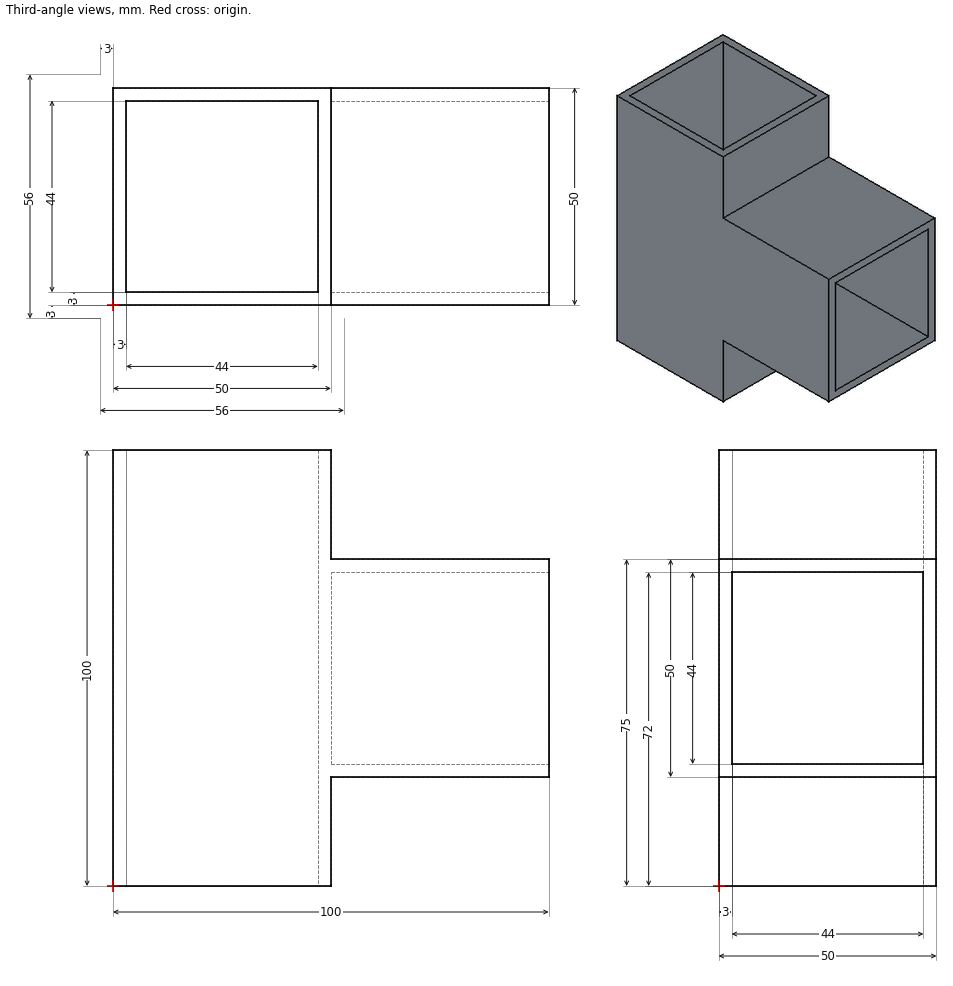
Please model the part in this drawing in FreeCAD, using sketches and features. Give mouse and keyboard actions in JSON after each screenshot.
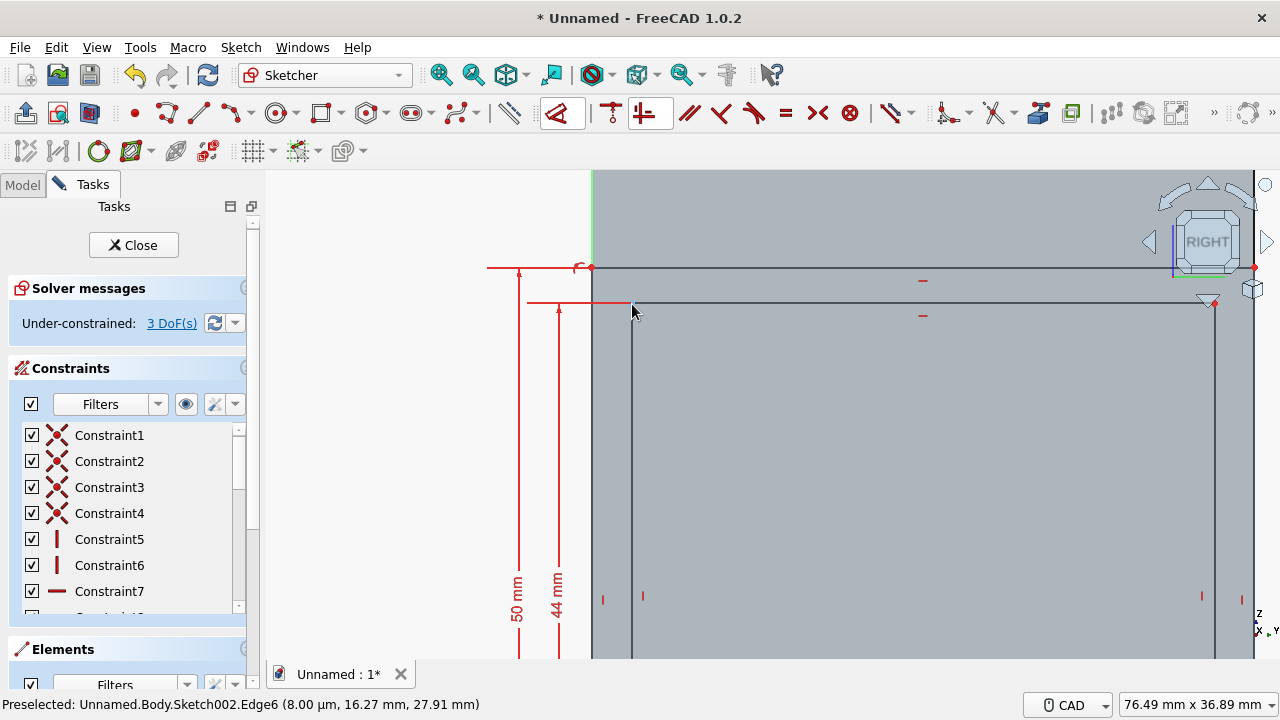
{"action": "left_click", "coordinate": [632, 303]}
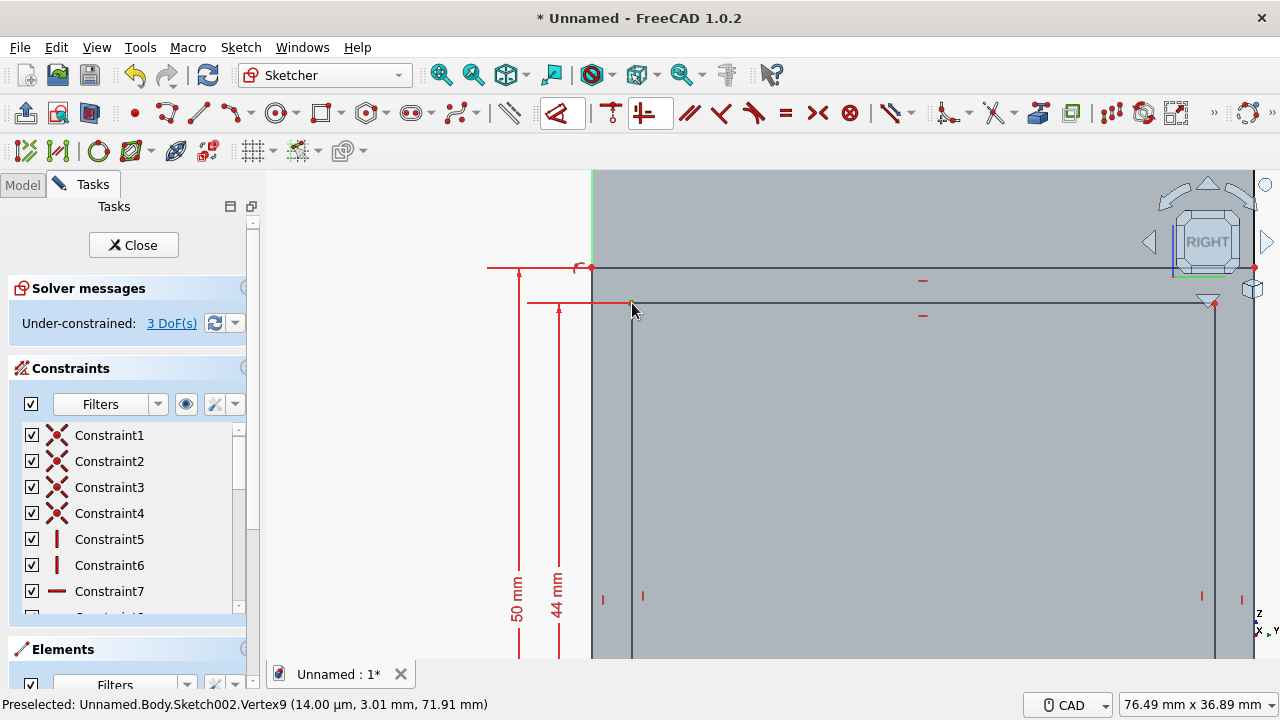
{"action": "key", "text": "l"}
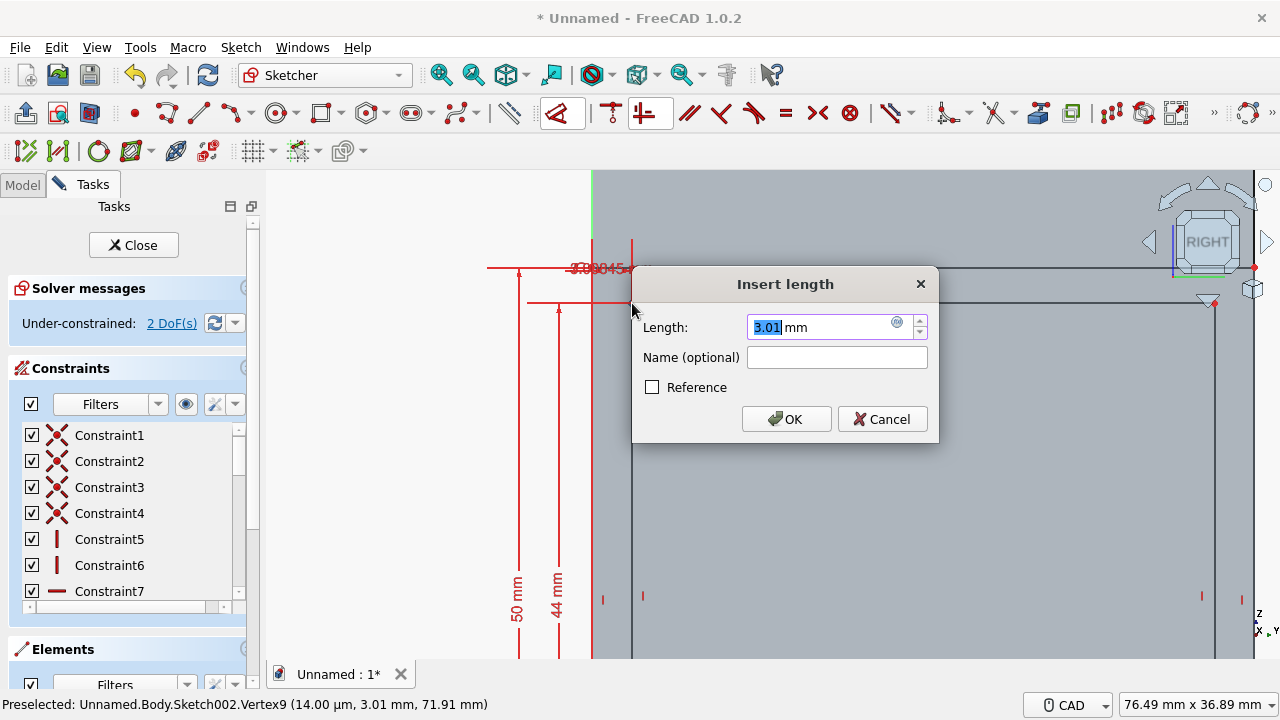
{"action": "type", "text": "3"}
{"action": "key", "text": "Return"}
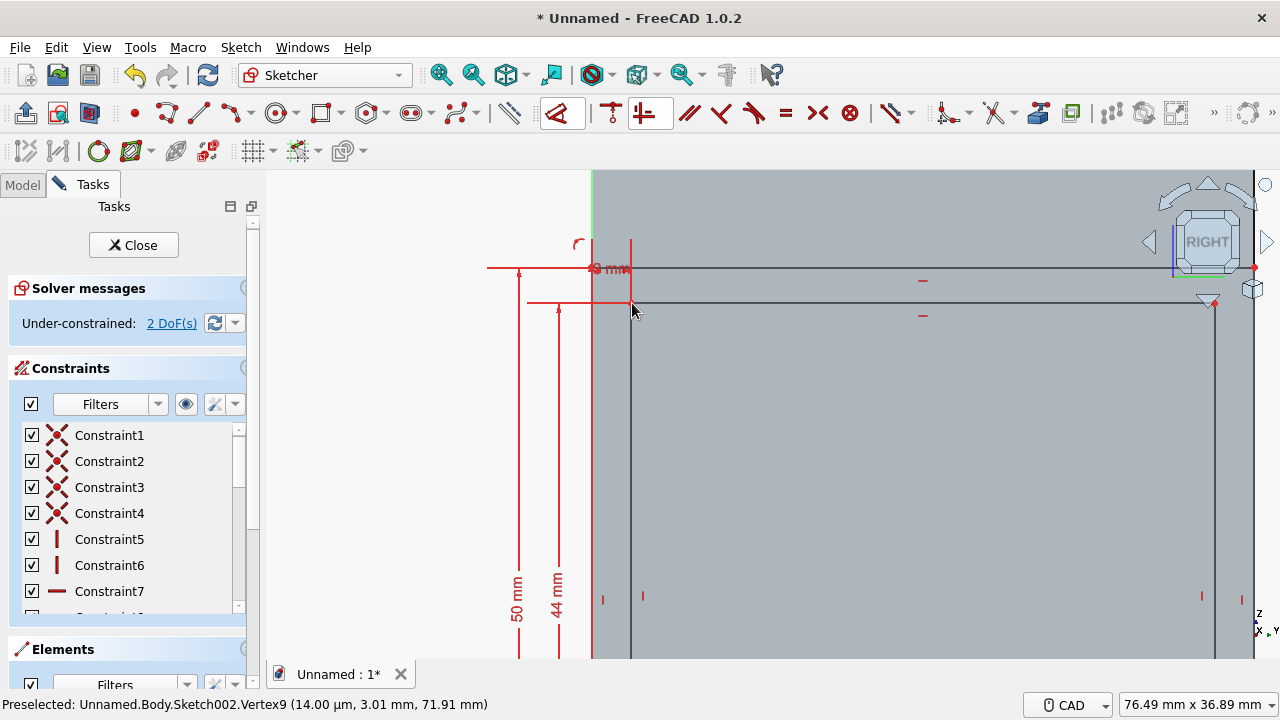
{"action": "scroll", "coordinate": [610, 266], "scroll_direction": "down", "scroll_amount": 6}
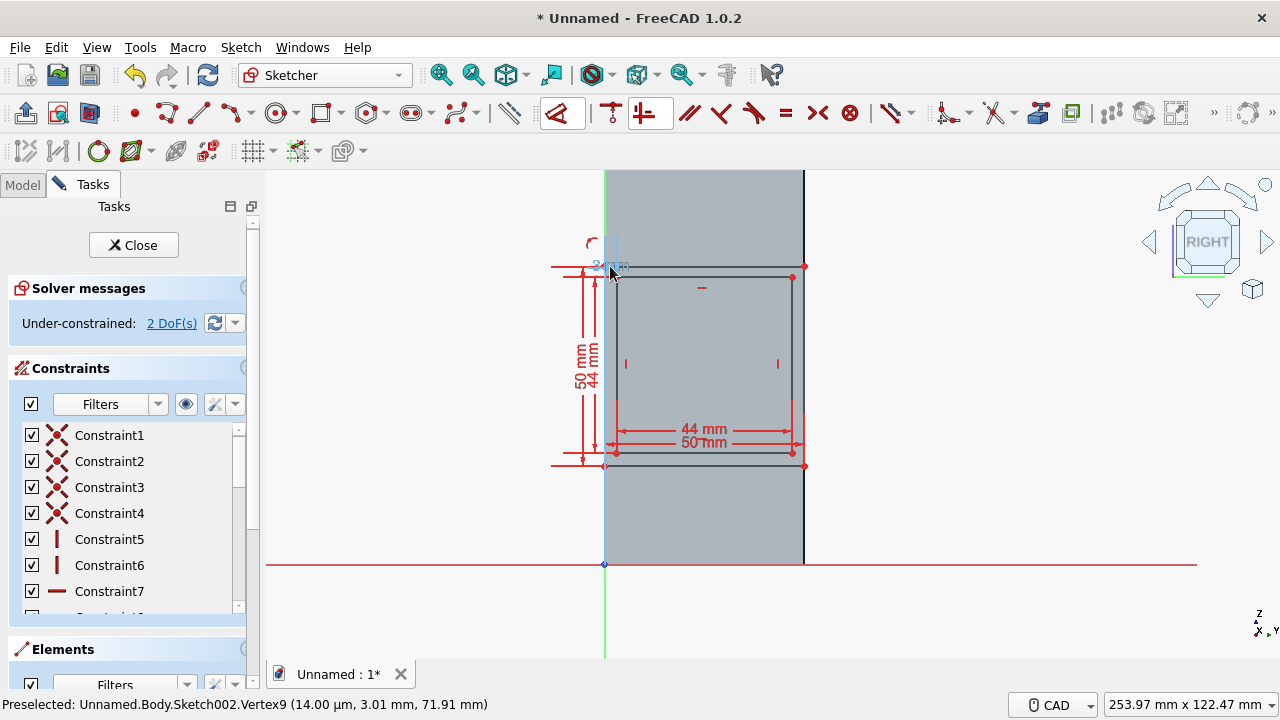
{"action": "left_click", "coordinate": [605, 267]}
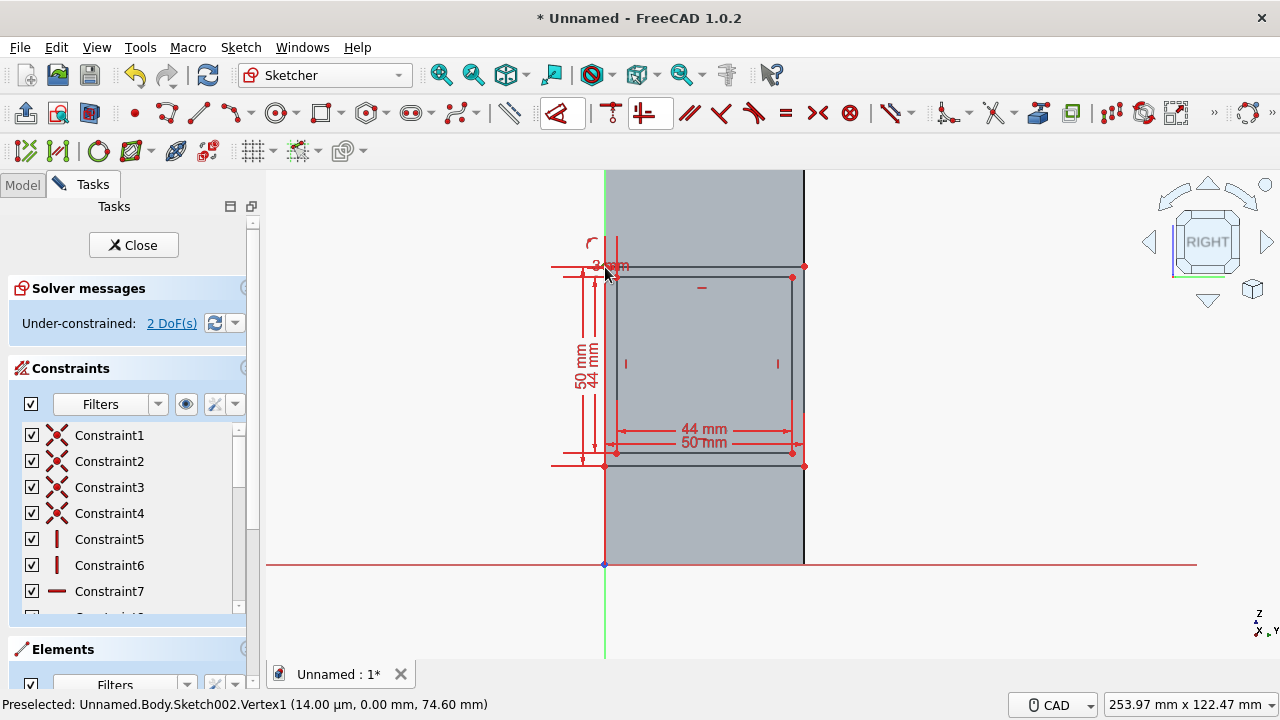
{"action": "key", "text": "i"}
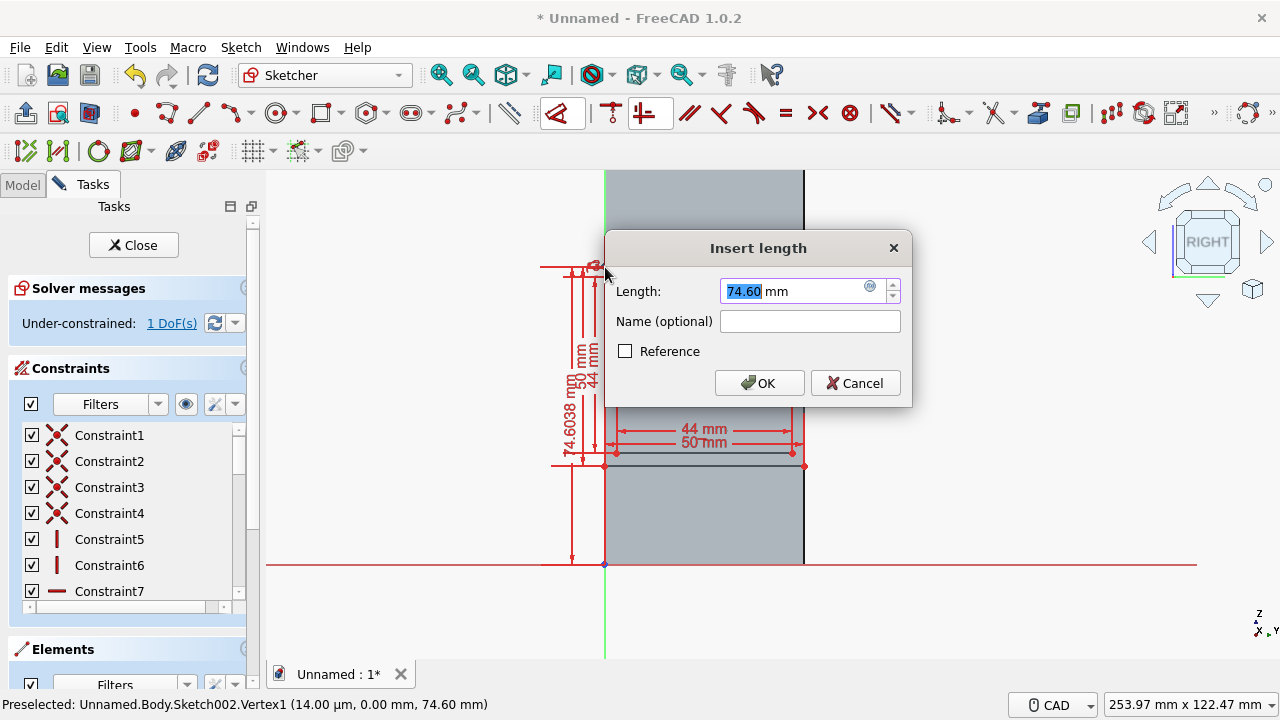
{"action": "type", "text": "75"}
{"action": "key", "text": "Return"}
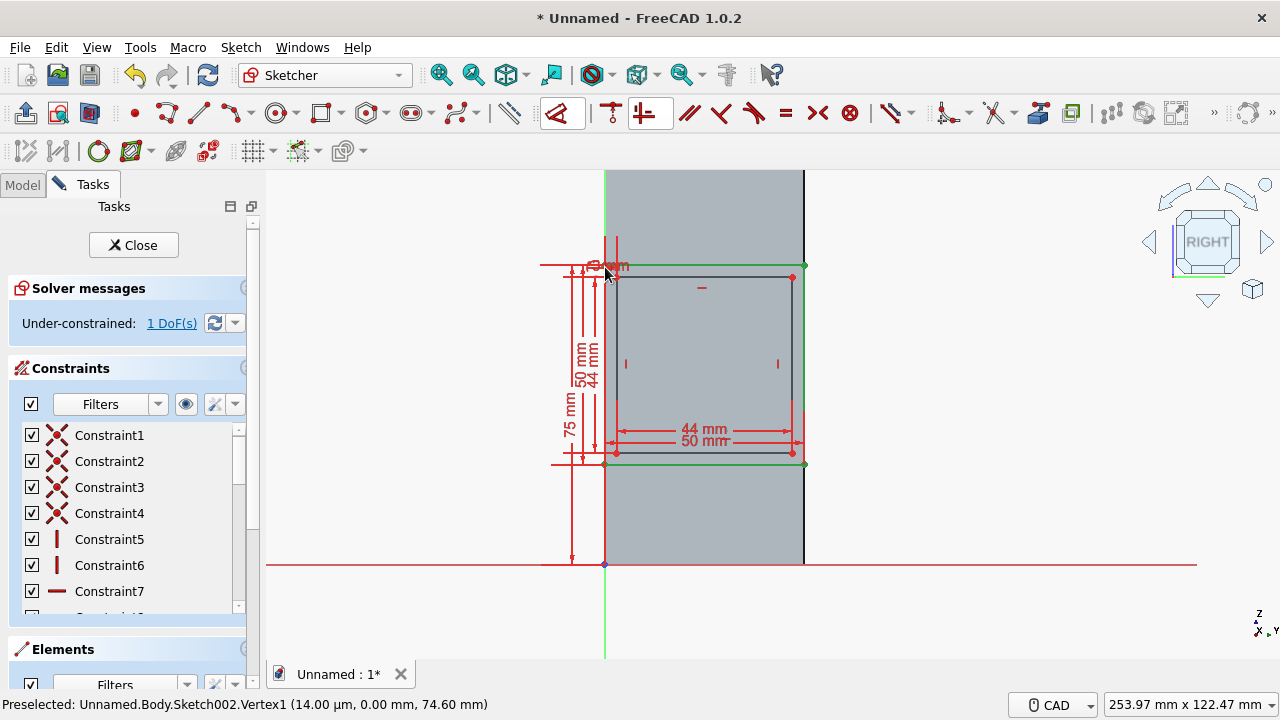
{"action": "left_click", "coordinate": [617, 277]}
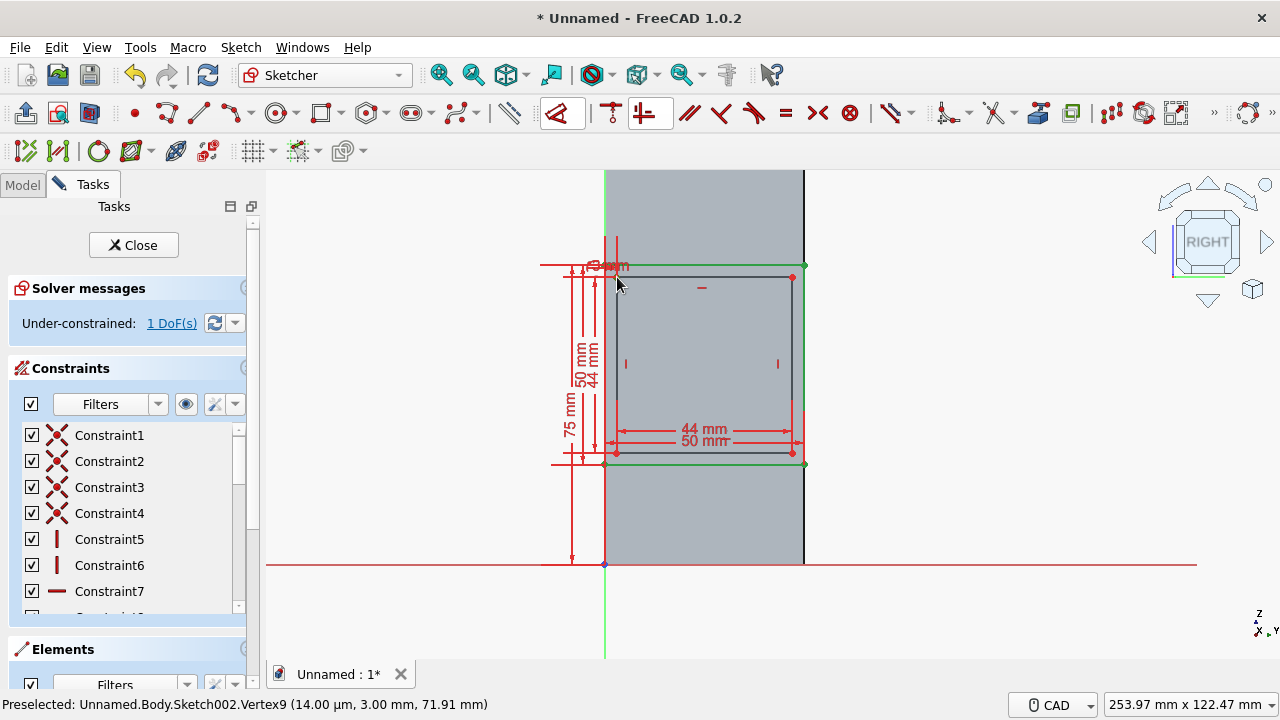
{"action": "key", "text": "i"}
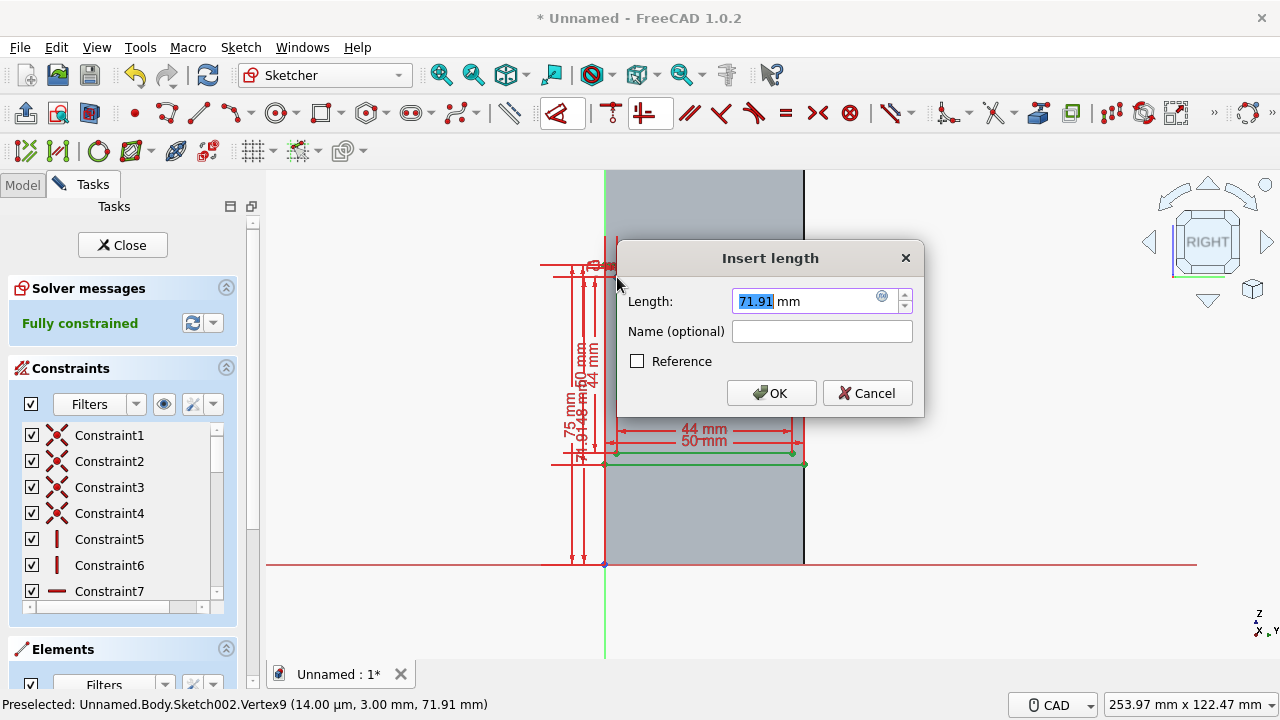
{"action": "type", "text": "72"}
{"action": "key", "text": "Return"}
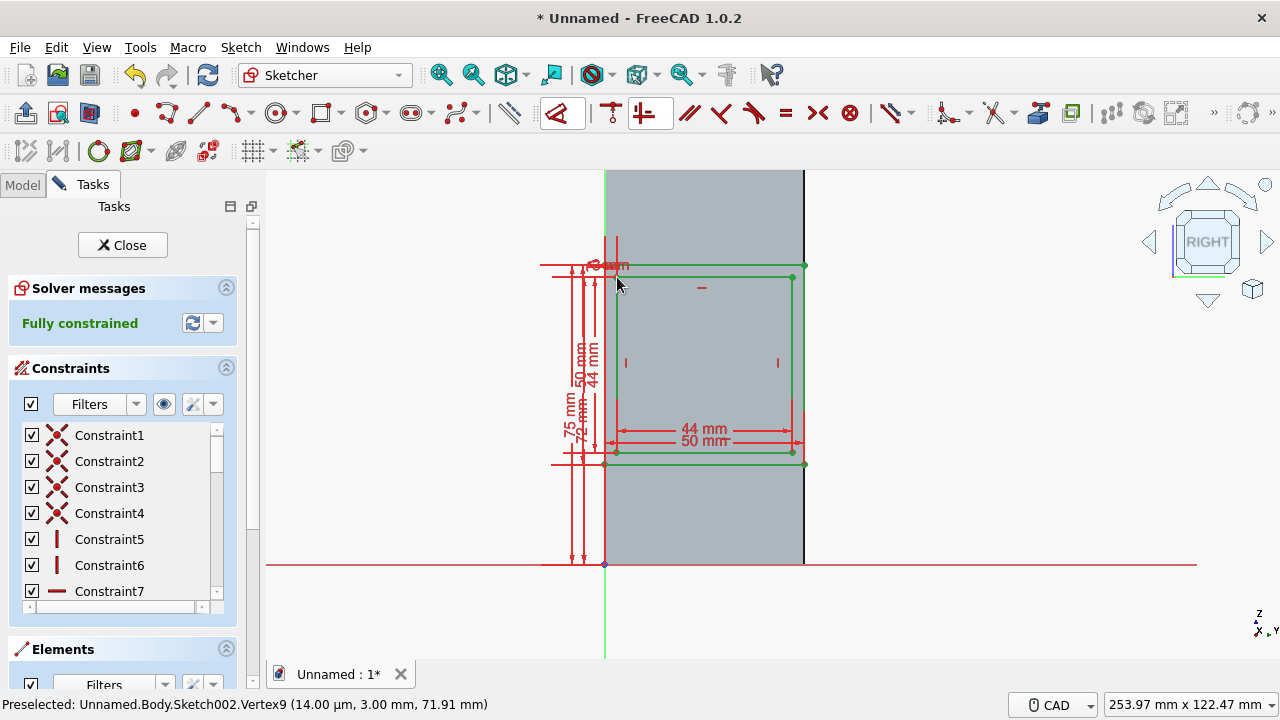
{"action": "left_click", "coordinate": [123, 245]}